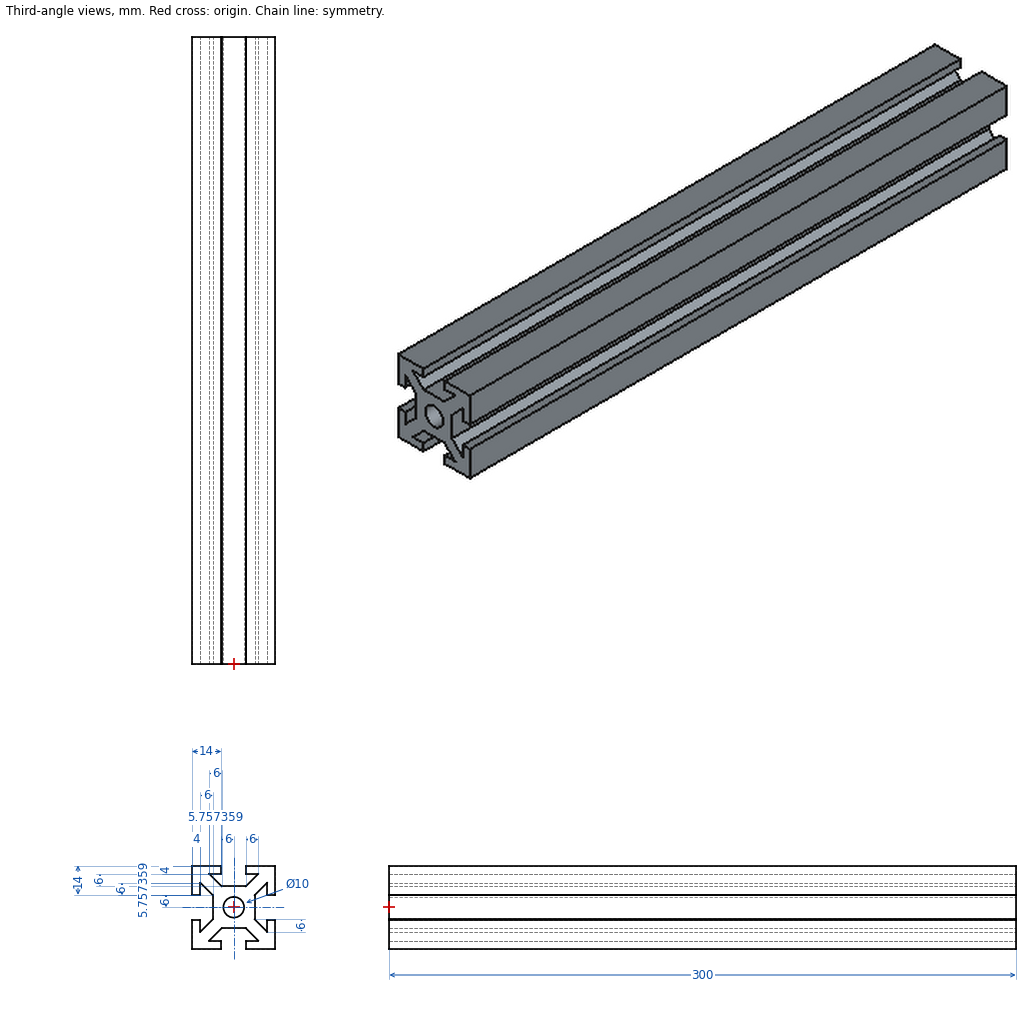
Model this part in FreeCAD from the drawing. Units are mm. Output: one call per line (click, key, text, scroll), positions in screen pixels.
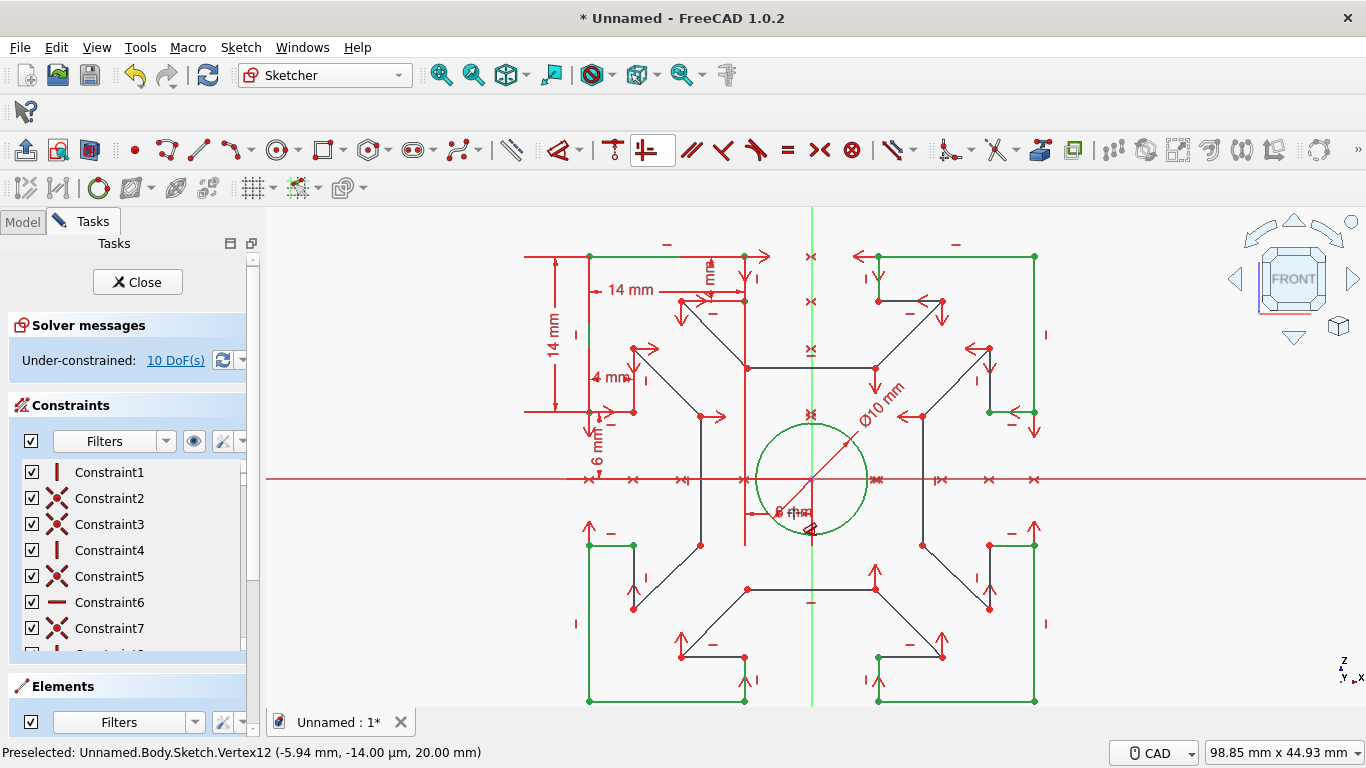
click(681, 396)
click(667, 315)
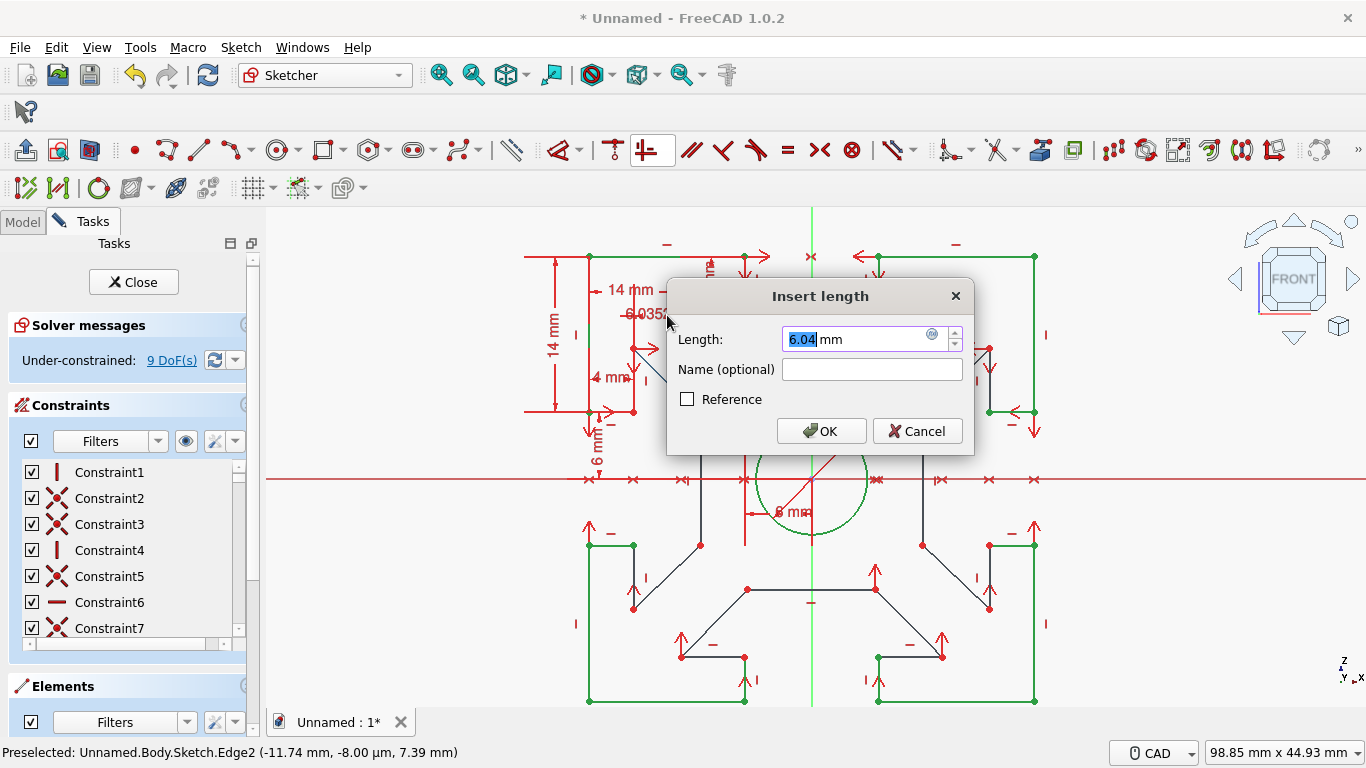
text(6)
key(Return)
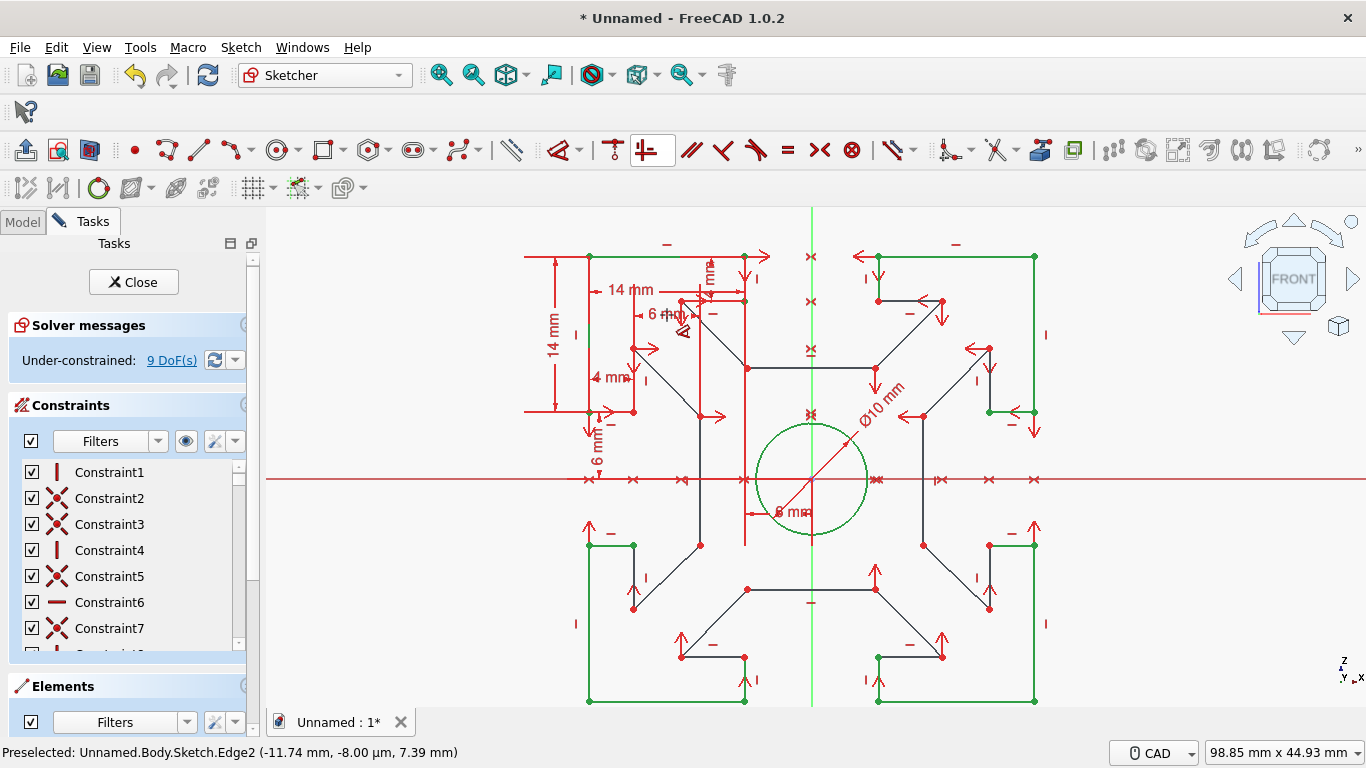
click(680, 396)
click(734, 383)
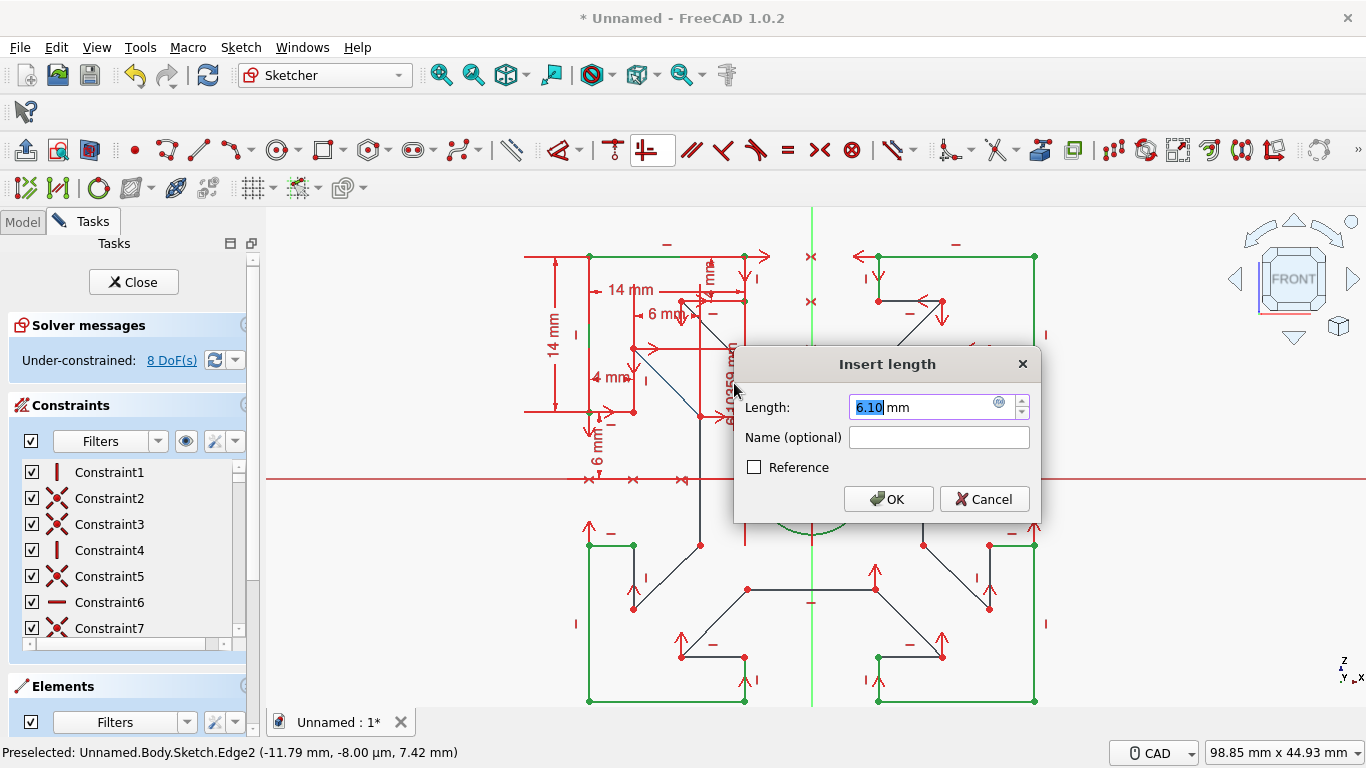
text(6)
key(Return)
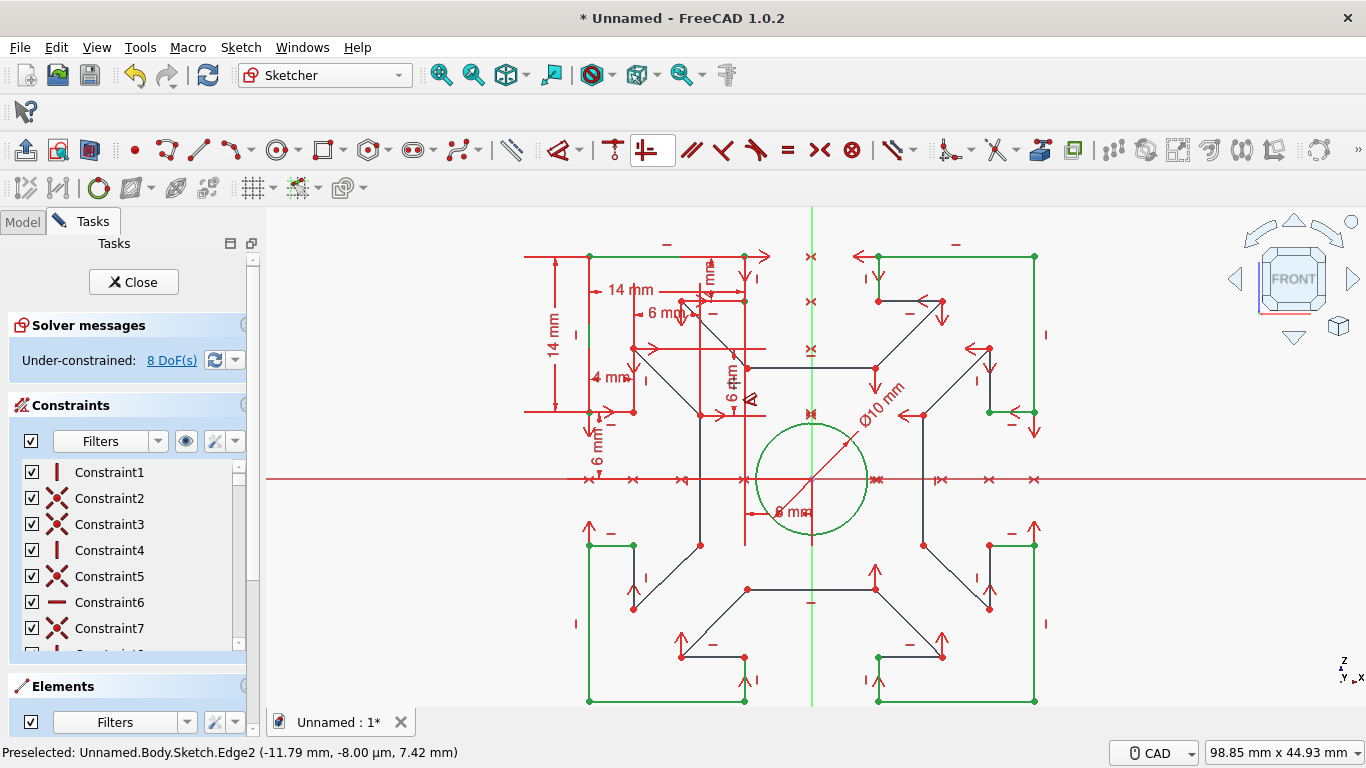
click(701, 321)
click(714, 243)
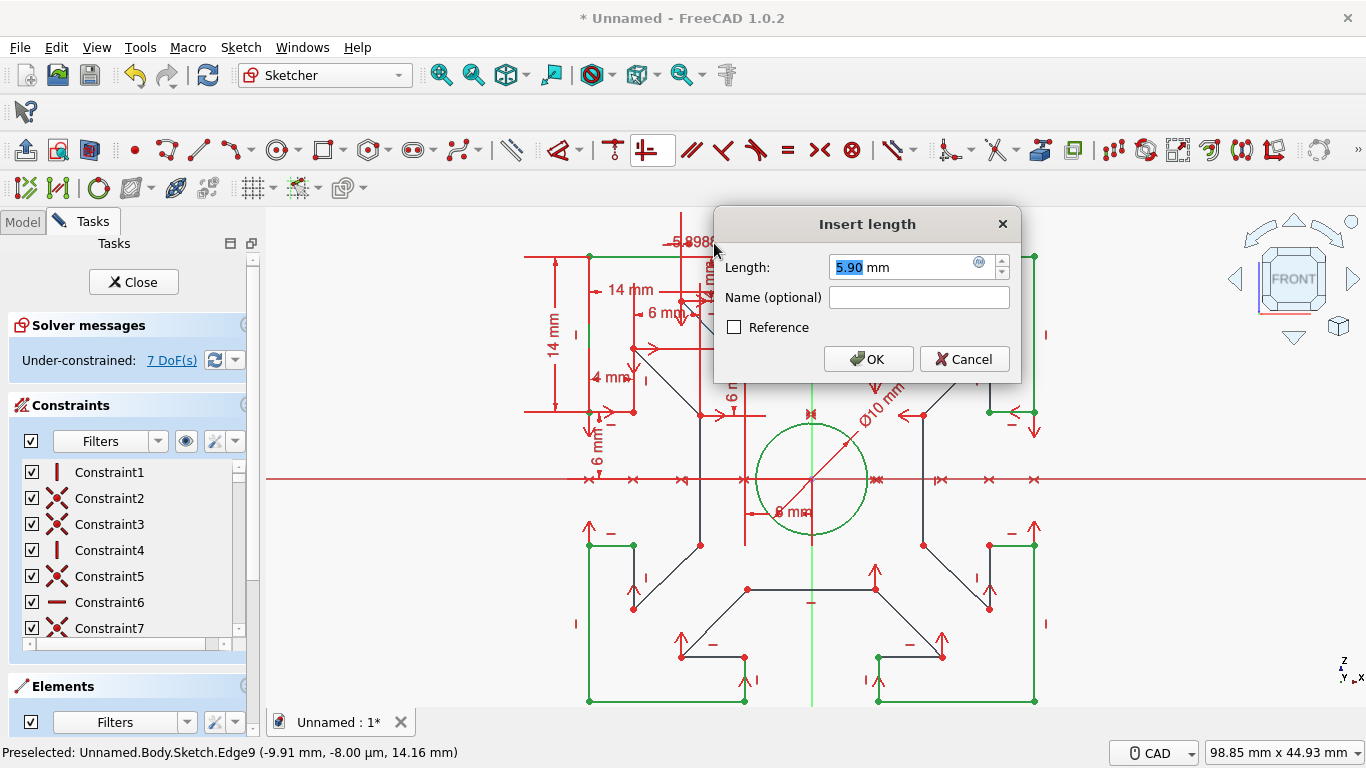
text(6)
key(Return)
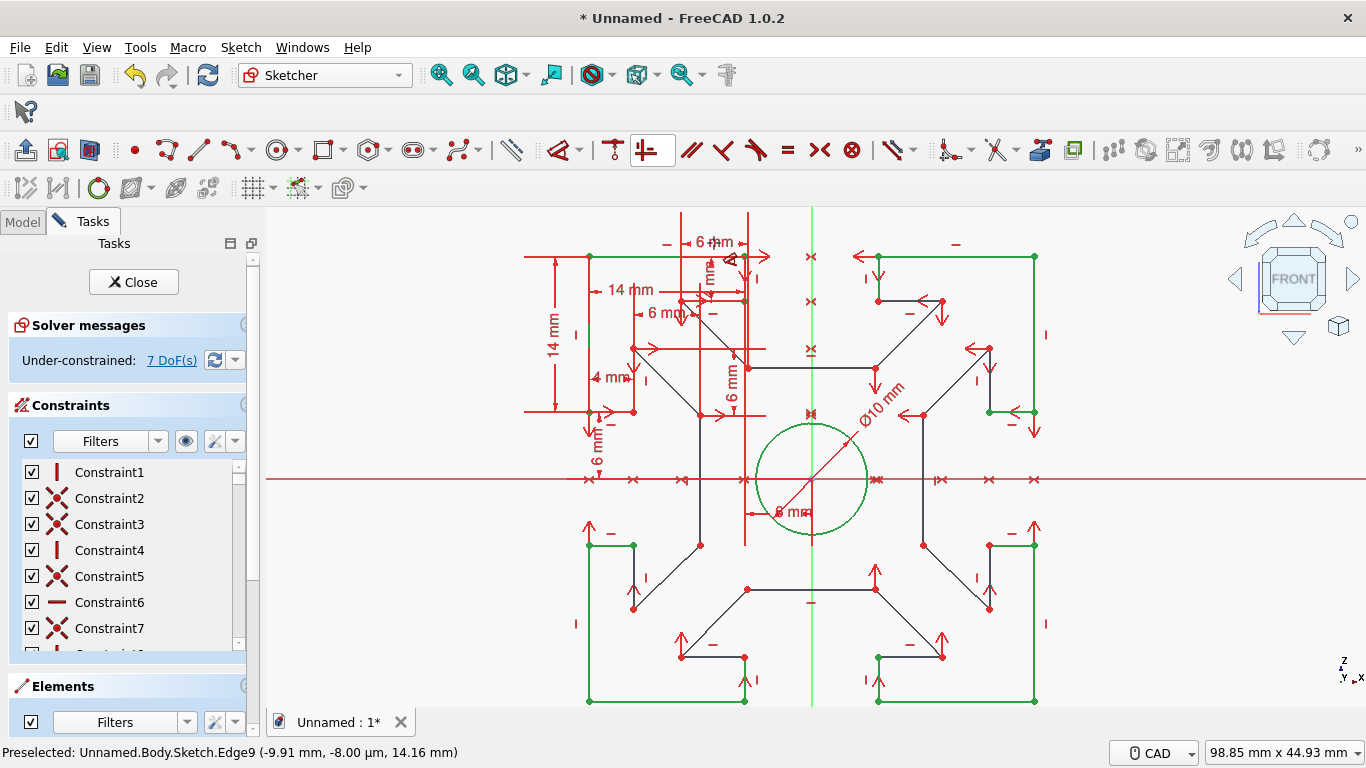
click(702, 321)
click(782, 335)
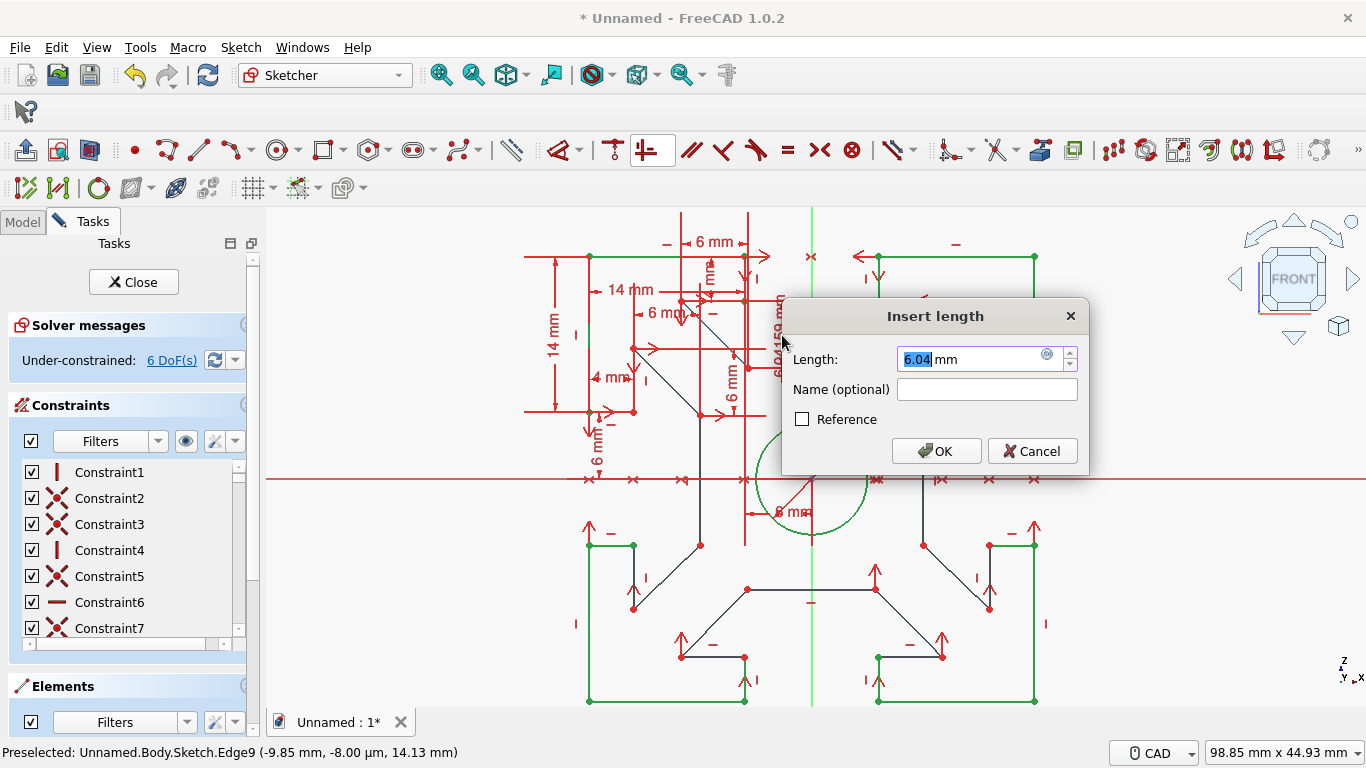
text(6)
key(Return)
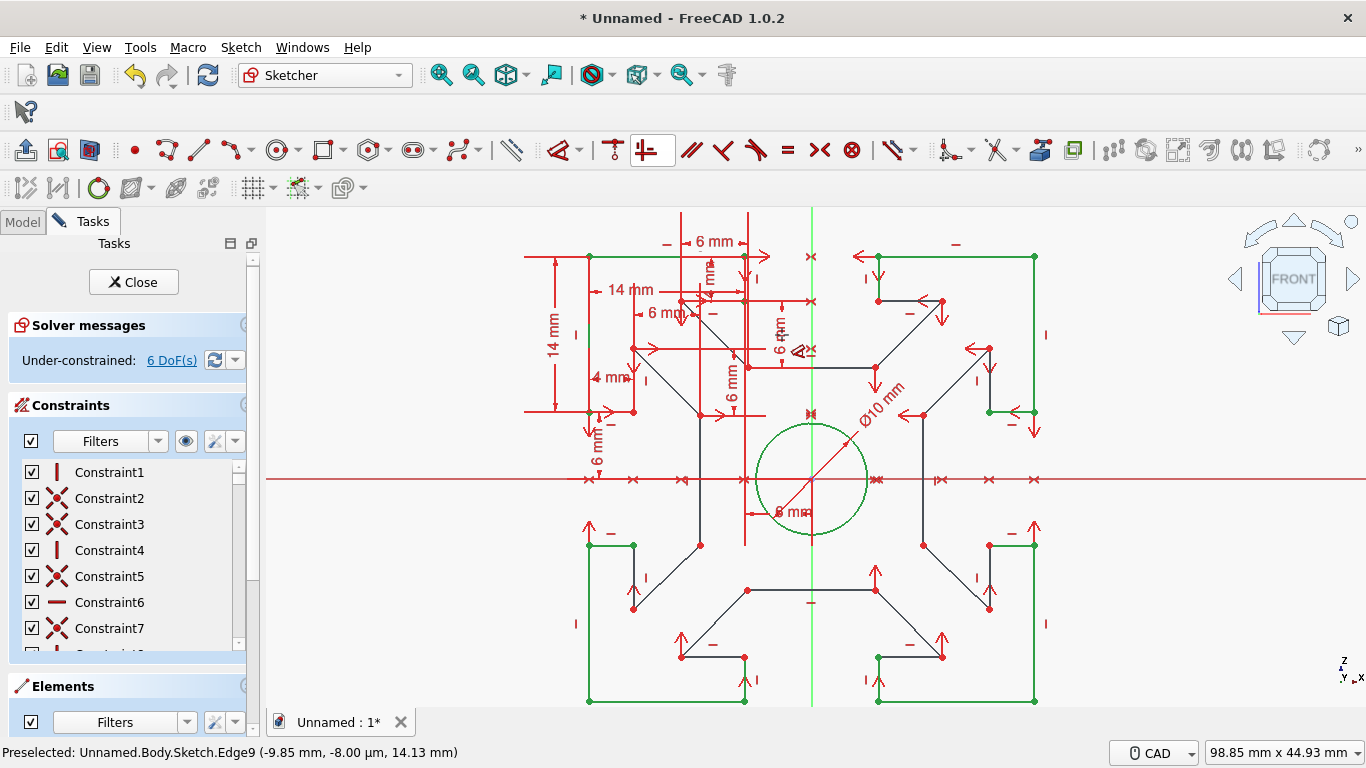
click(895, 348)
click(909, 243)